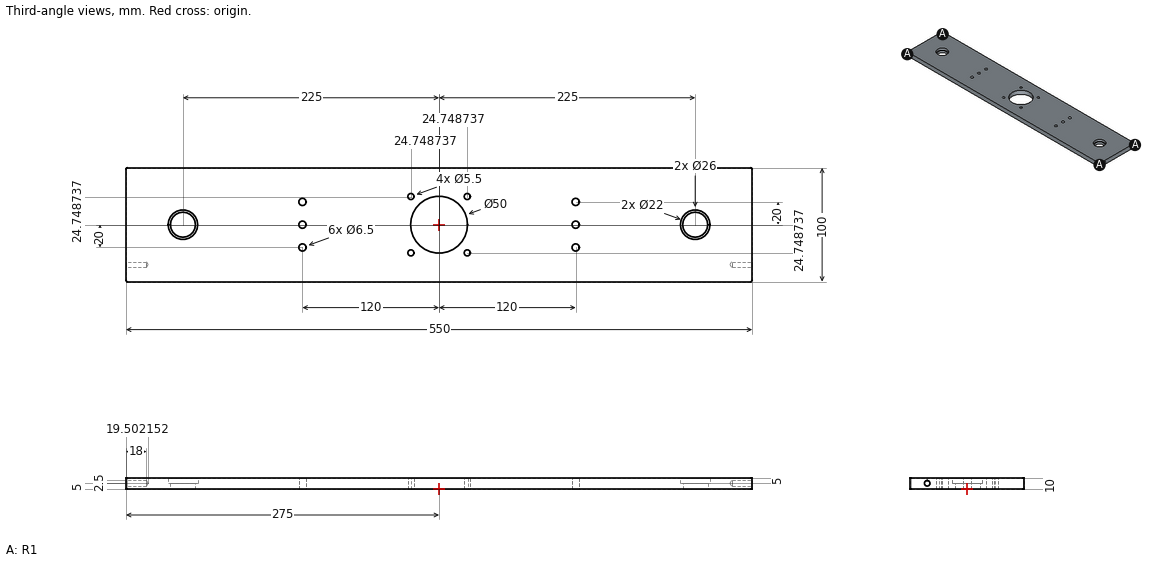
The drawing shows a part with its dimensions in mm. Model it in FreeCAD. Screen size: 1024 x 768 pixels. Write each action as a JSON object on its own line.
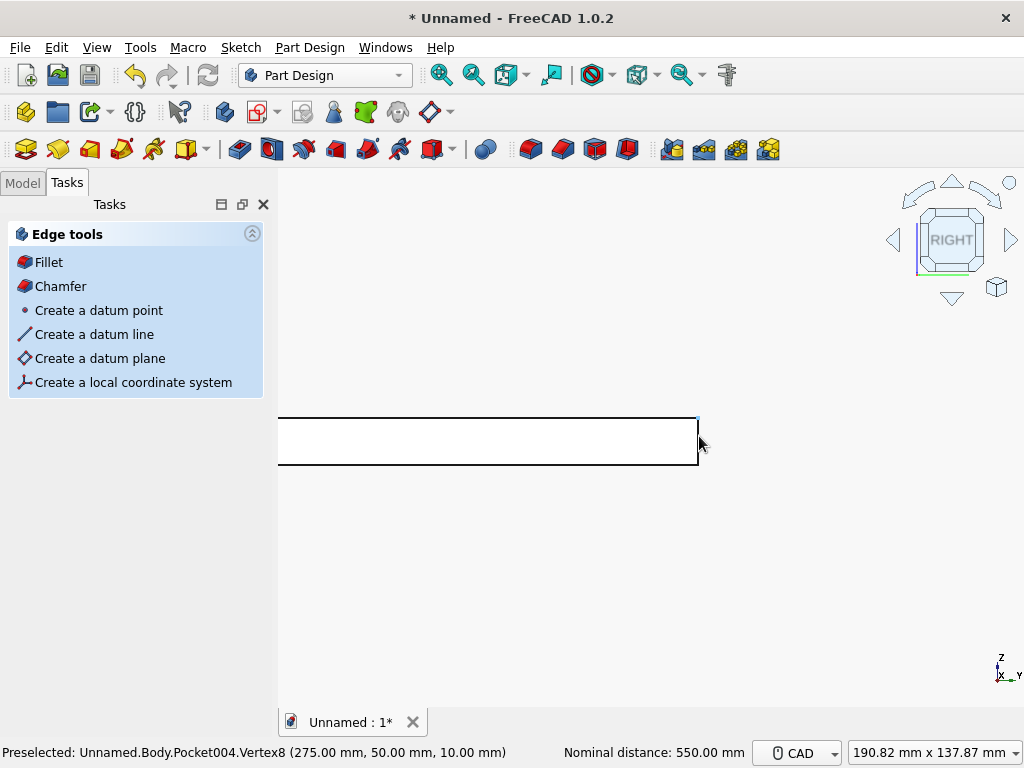
{"action": "left_click", "coordinate": [698, 440], "text": "ctrl"}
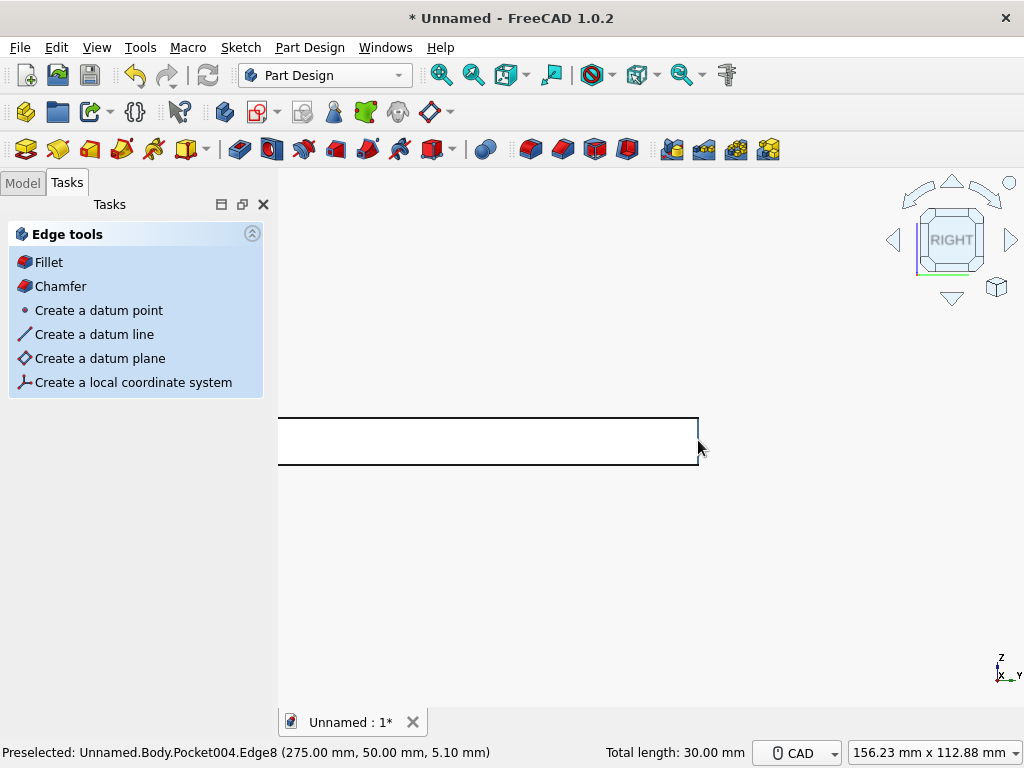
{"action": "key", "text": "v f"}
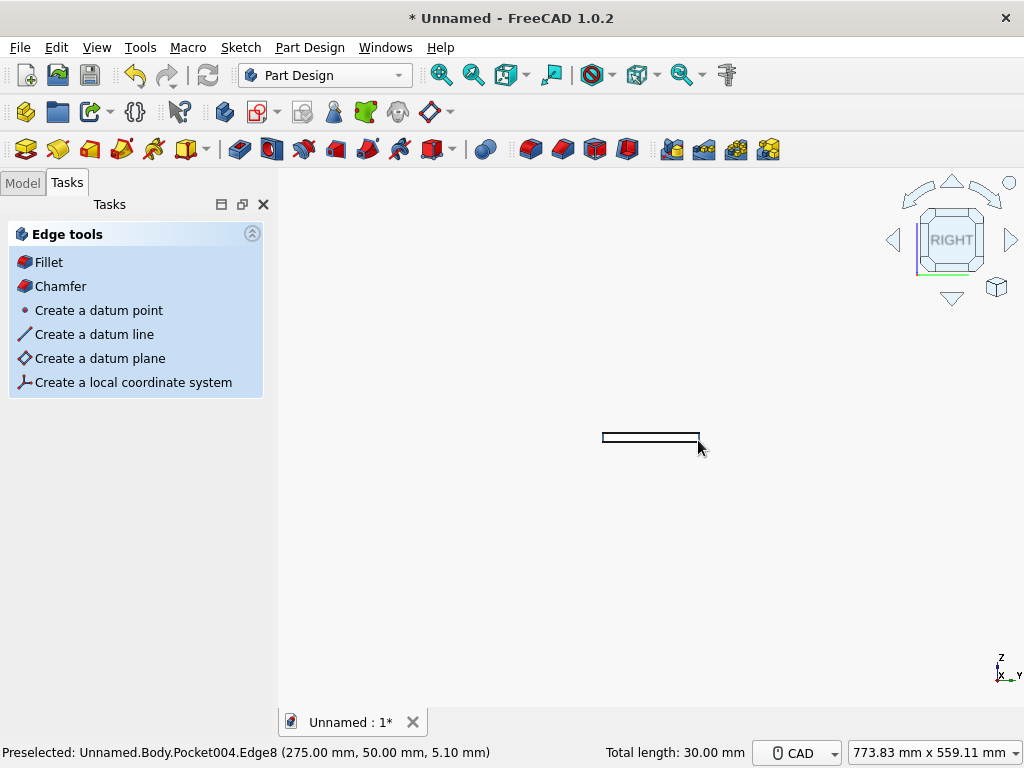
{"action": "key", "text": "5"}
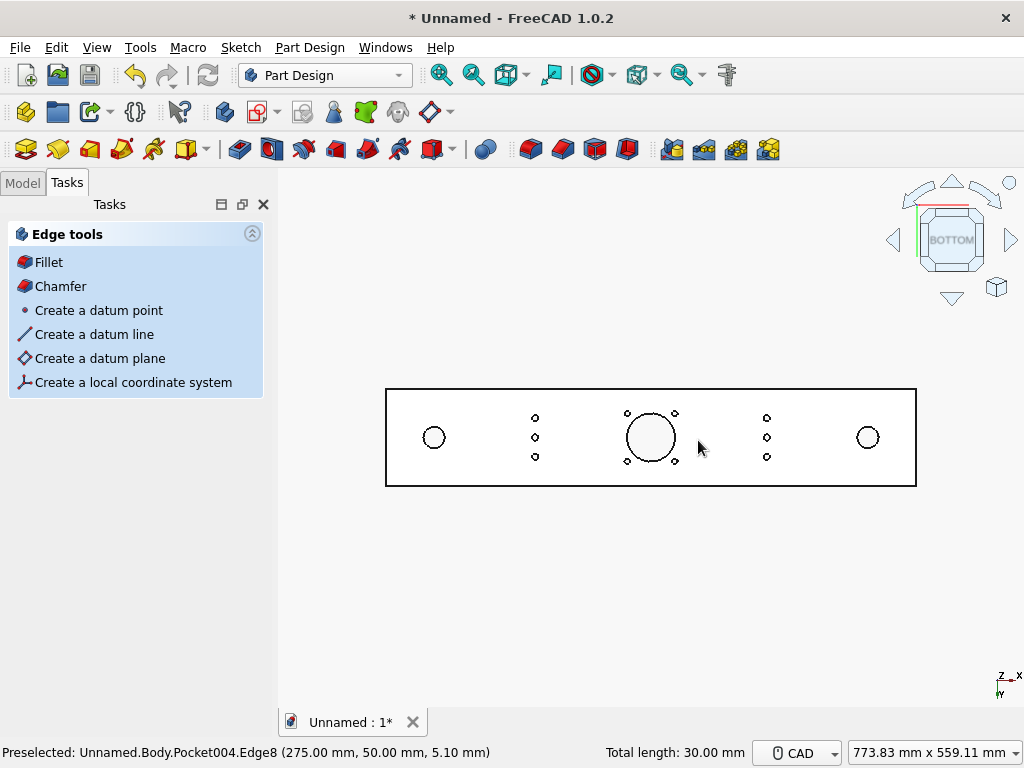
{"action": "scroll", "coordinate": [386, 485], "scroll_direction": "up", "scroll_amount": 8}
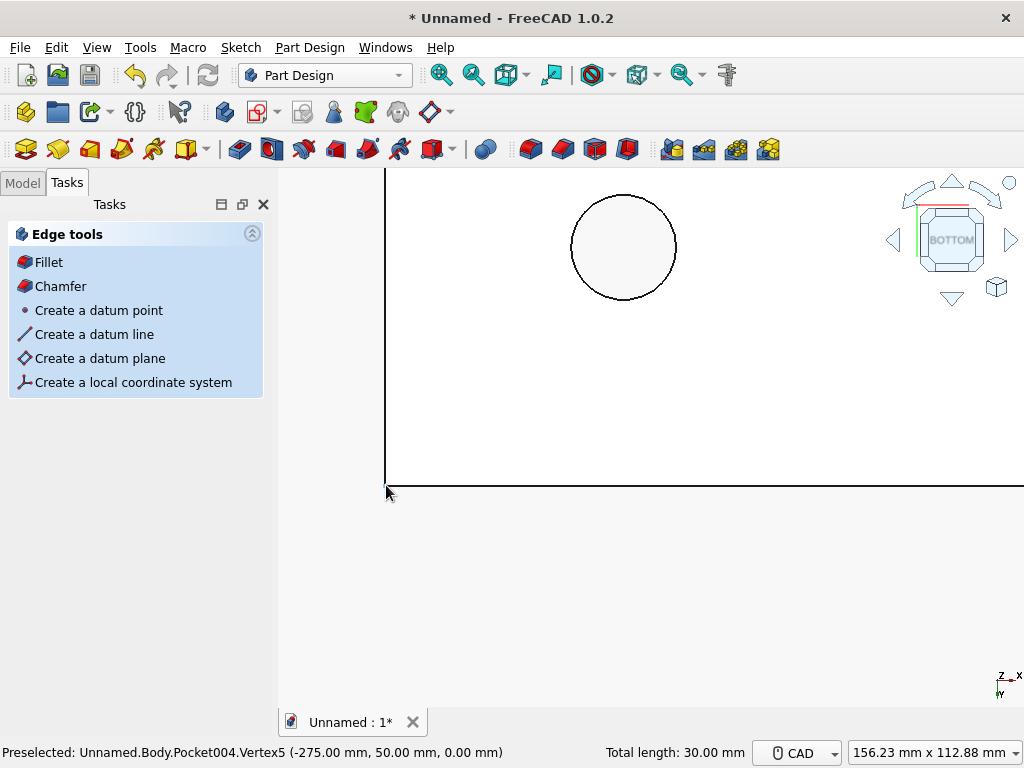
{"action": "key", "text": "v f"}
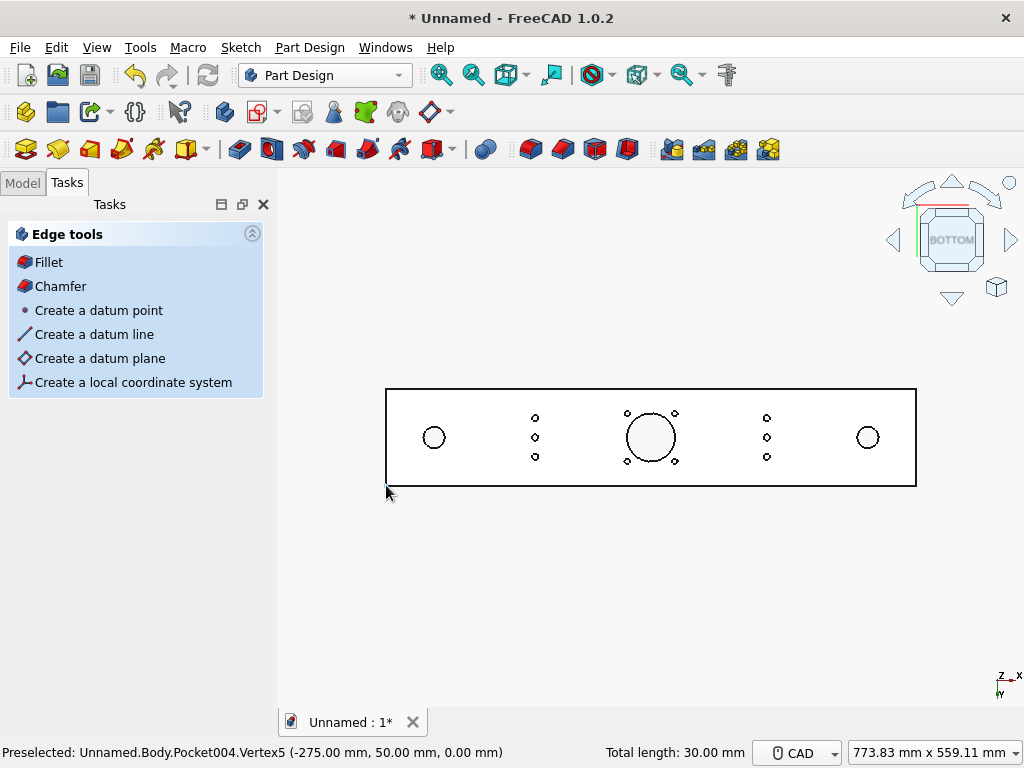
{"action": "key", "text": "4"}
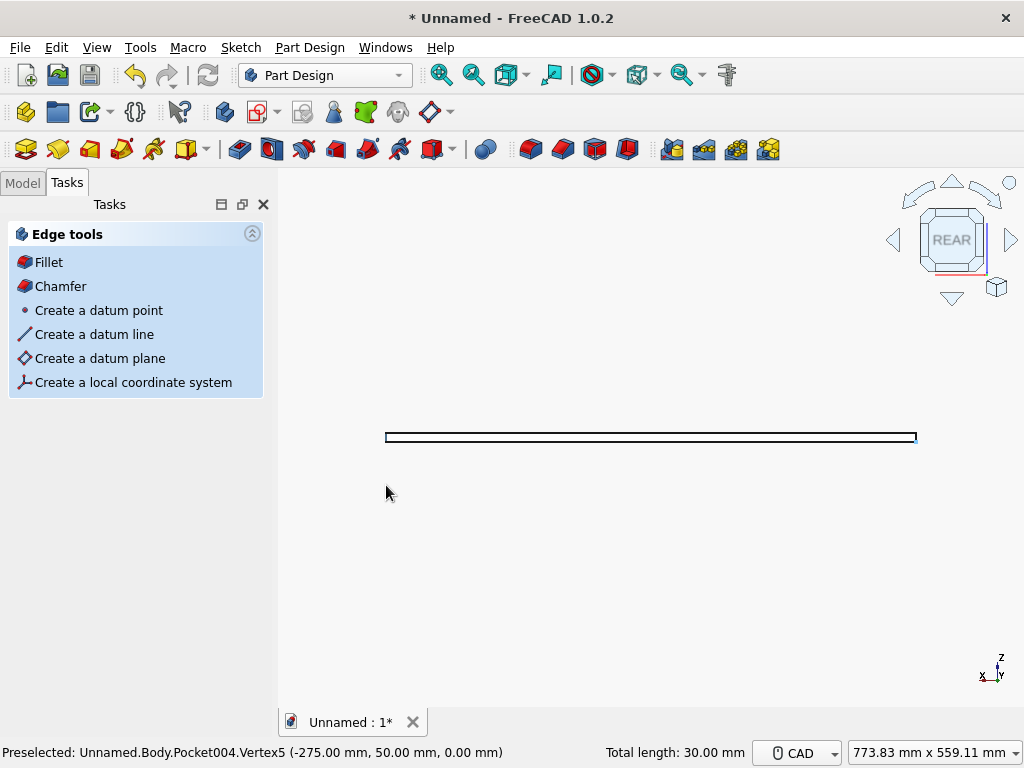
{"action": "key", "text": "6"}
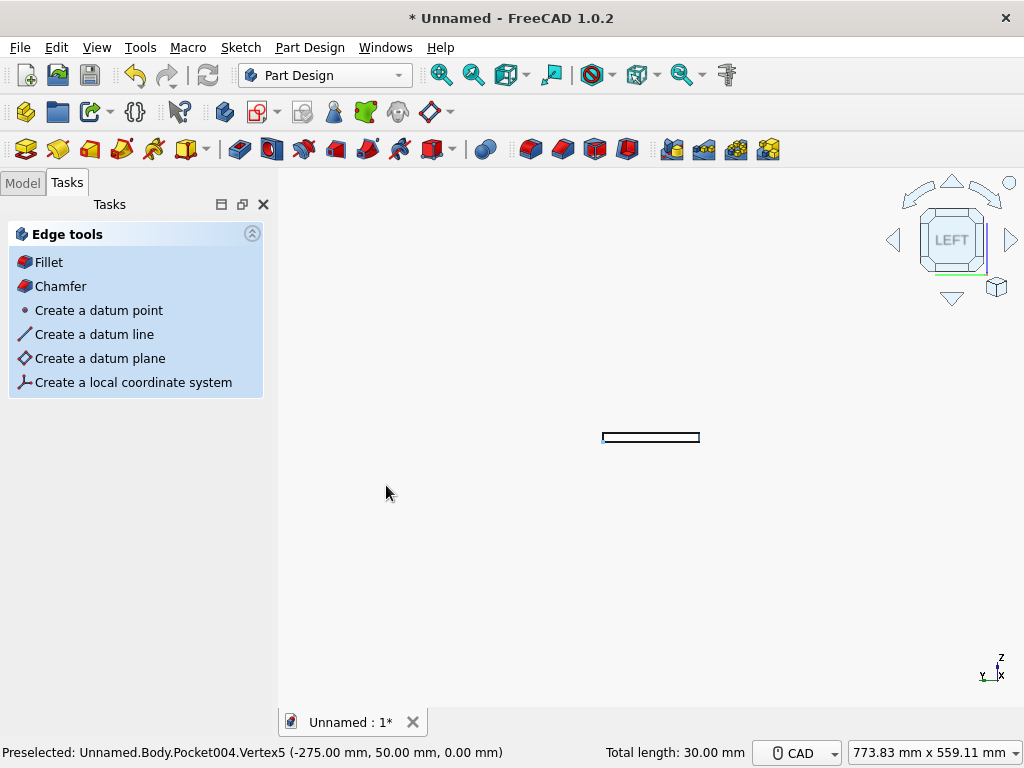
{"action": "key", "text": "v f"}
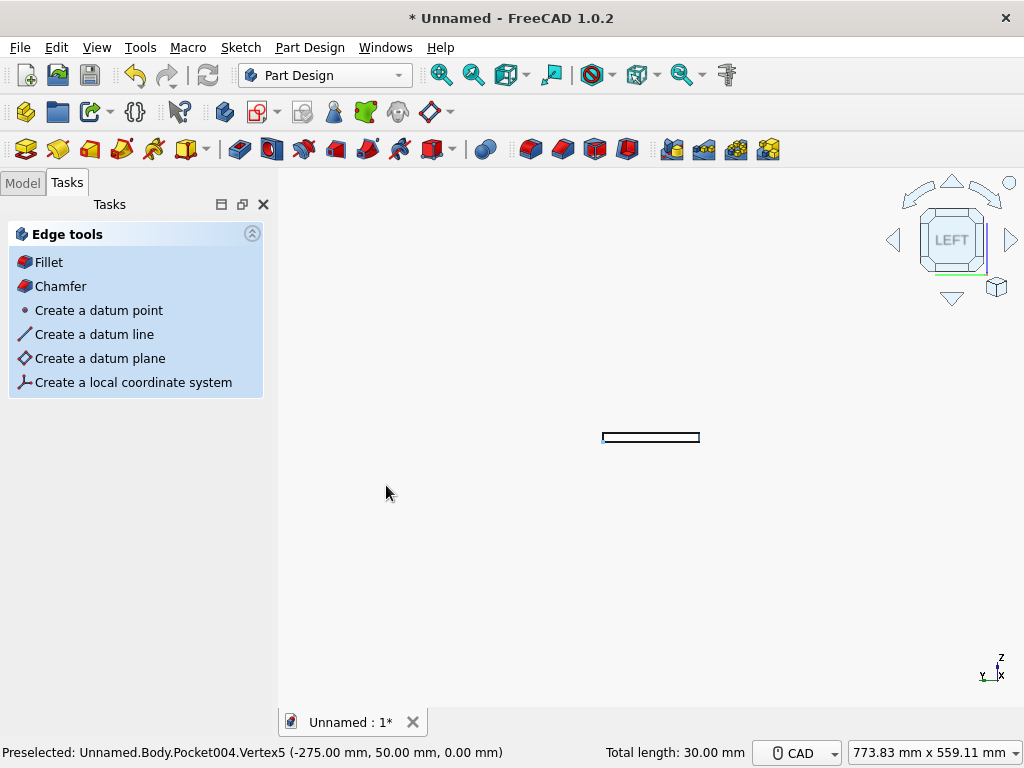
{"action": "scroll", "coordinate": [603, 436], "scroll_direction": "up", "scroll_amount": 8}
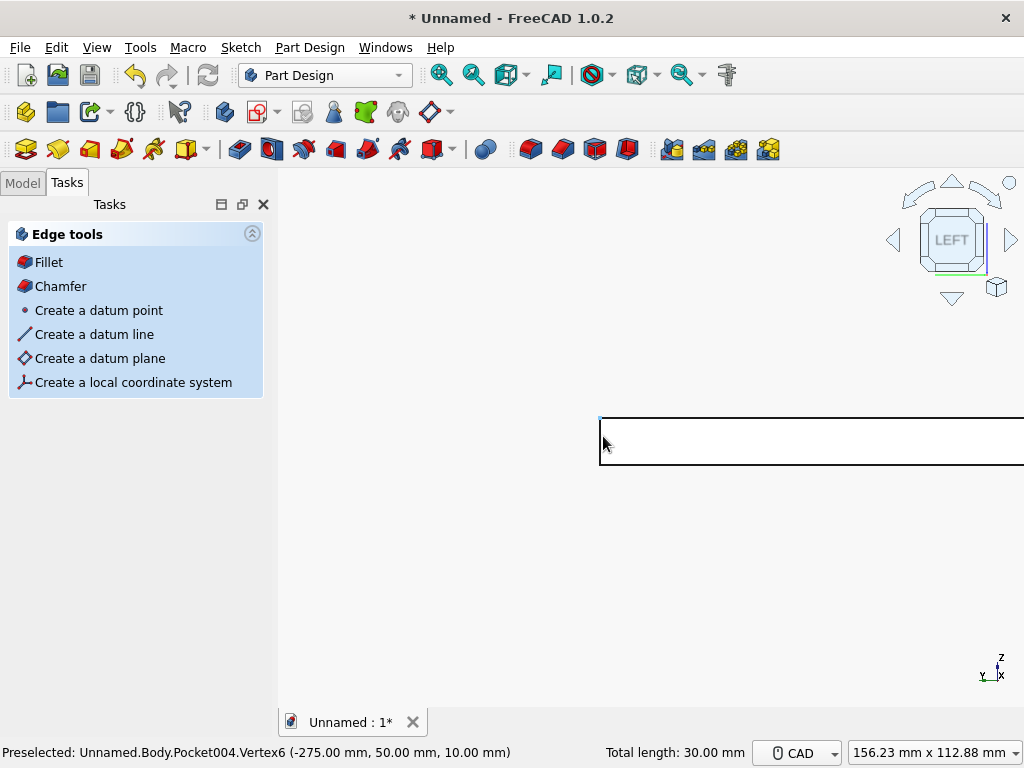
{"action": "left_click", "coordinate": [600, 440], "text": "ctrl"}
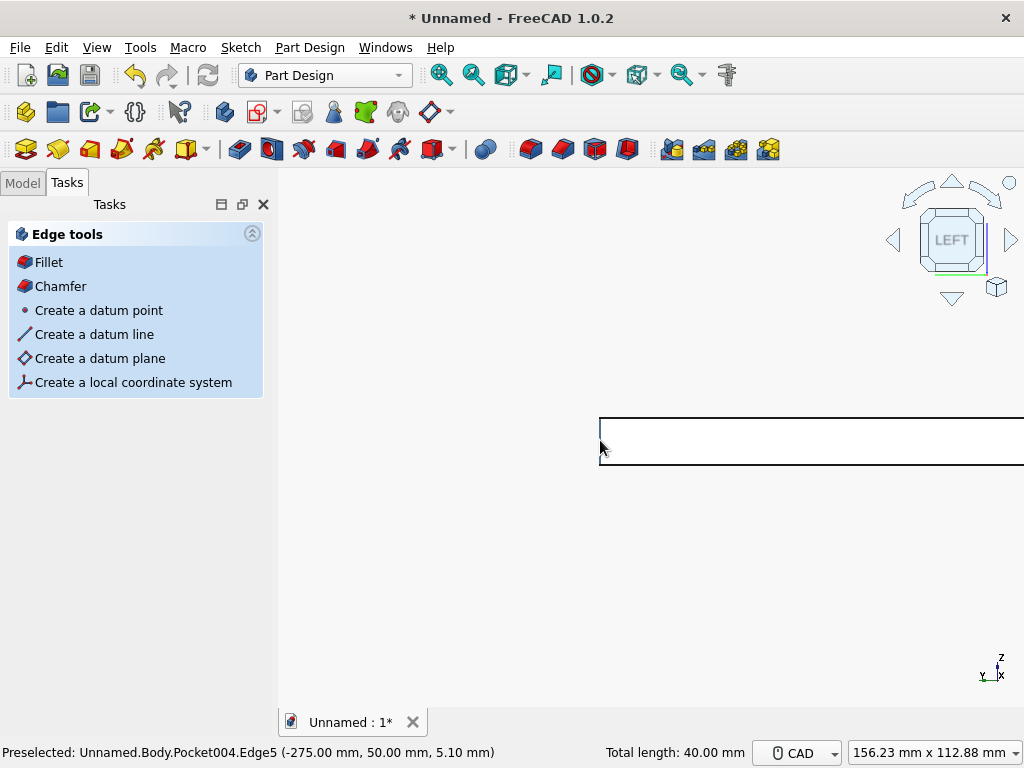
{"action": "left_click", "coordinate": [532, 150]}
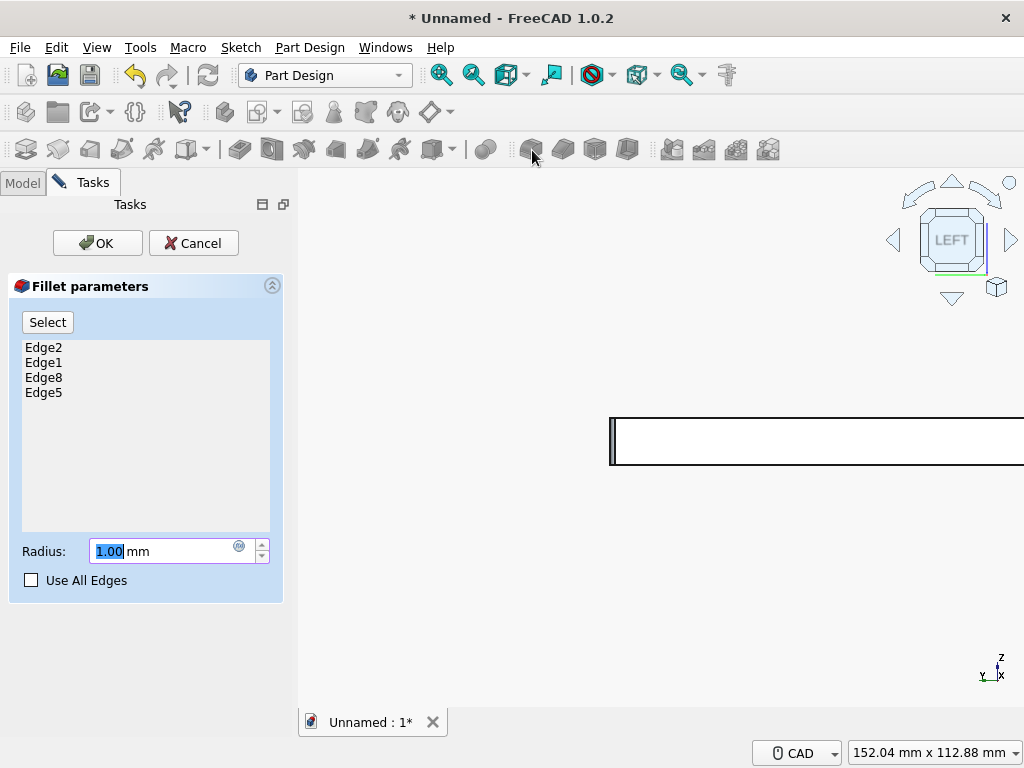
{"action": "type", "text": "1"}
{"action": "key", "text": "Tab"}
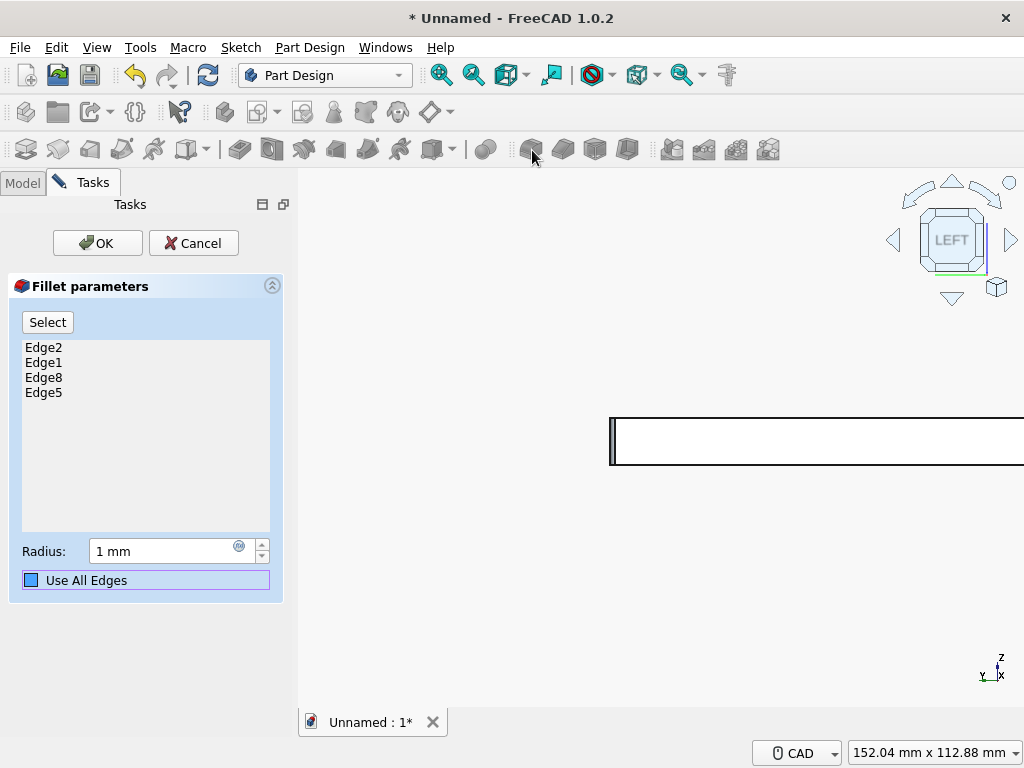
{"action": "left_click", "coordinate": [98, 243]}